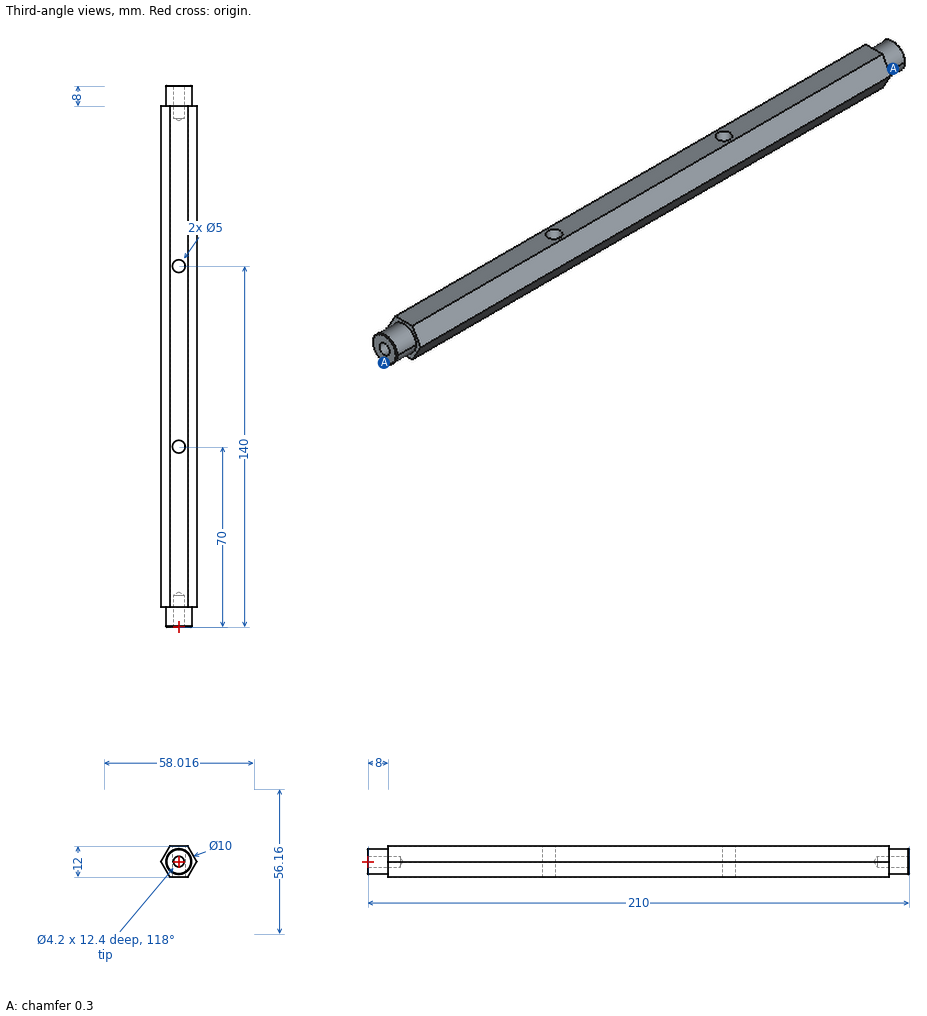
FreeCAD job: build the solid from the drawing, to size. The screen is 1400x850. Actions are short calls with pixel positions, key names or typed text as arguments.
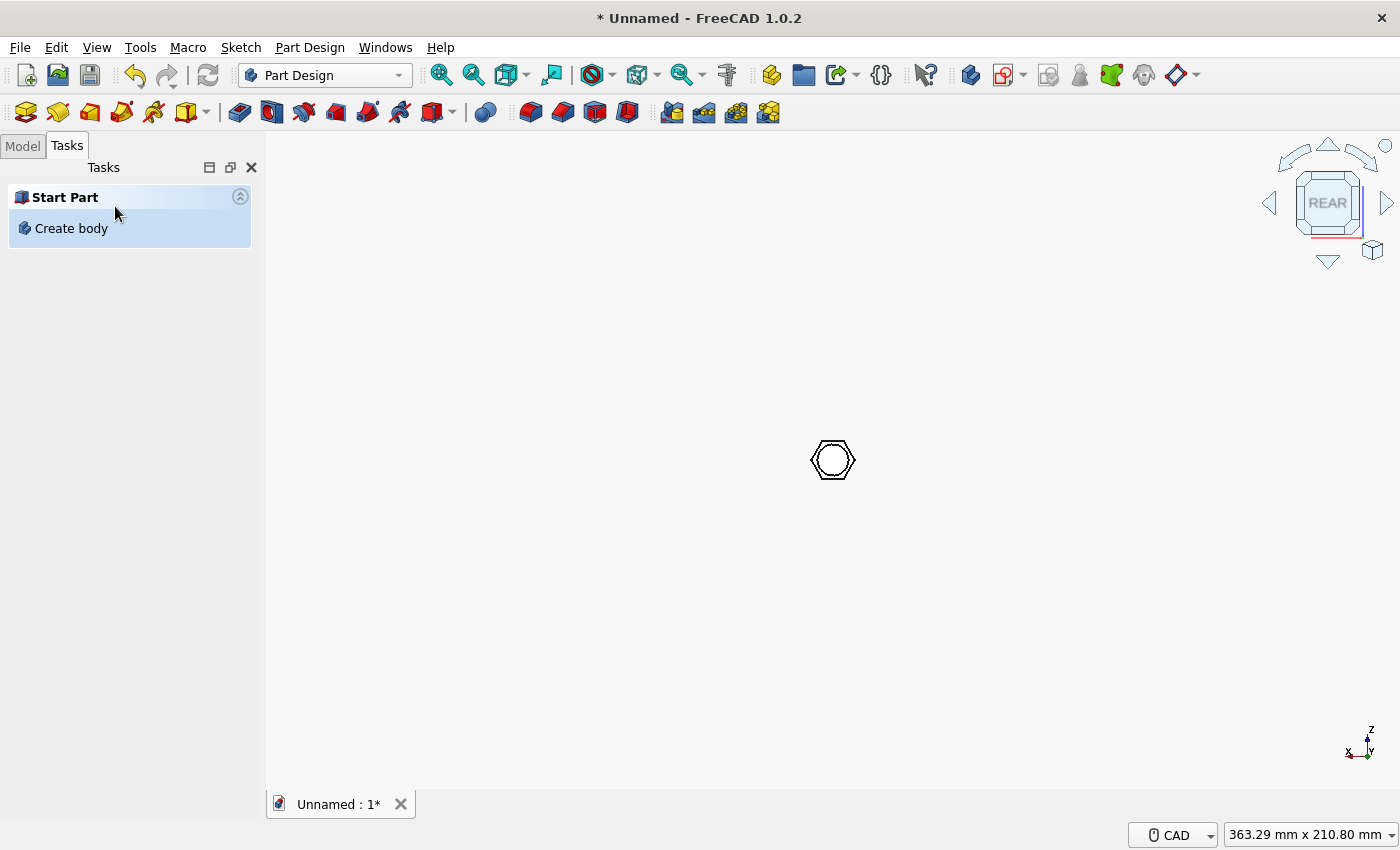
key(5)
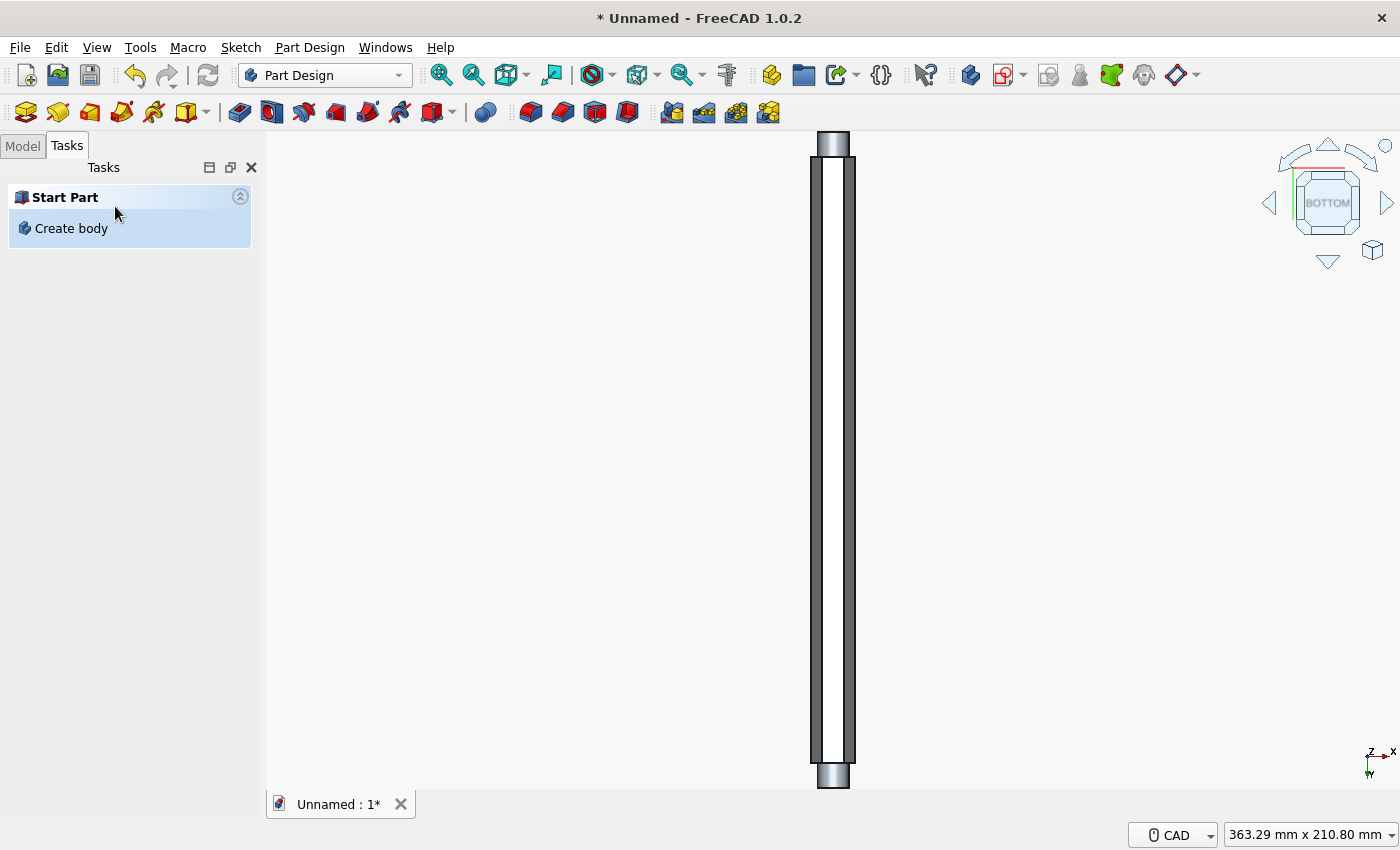
click(833, 719)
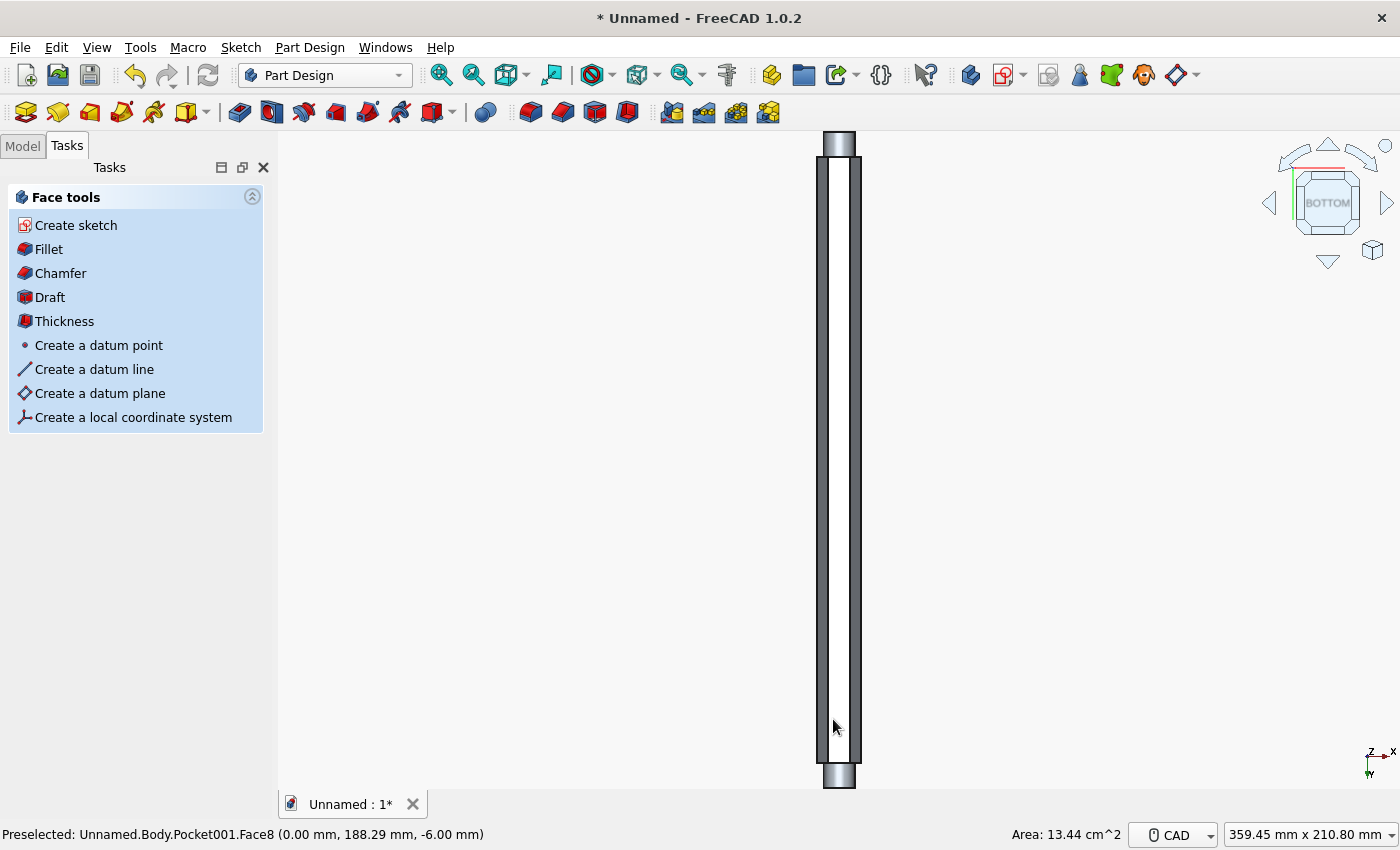
click(1004, 76)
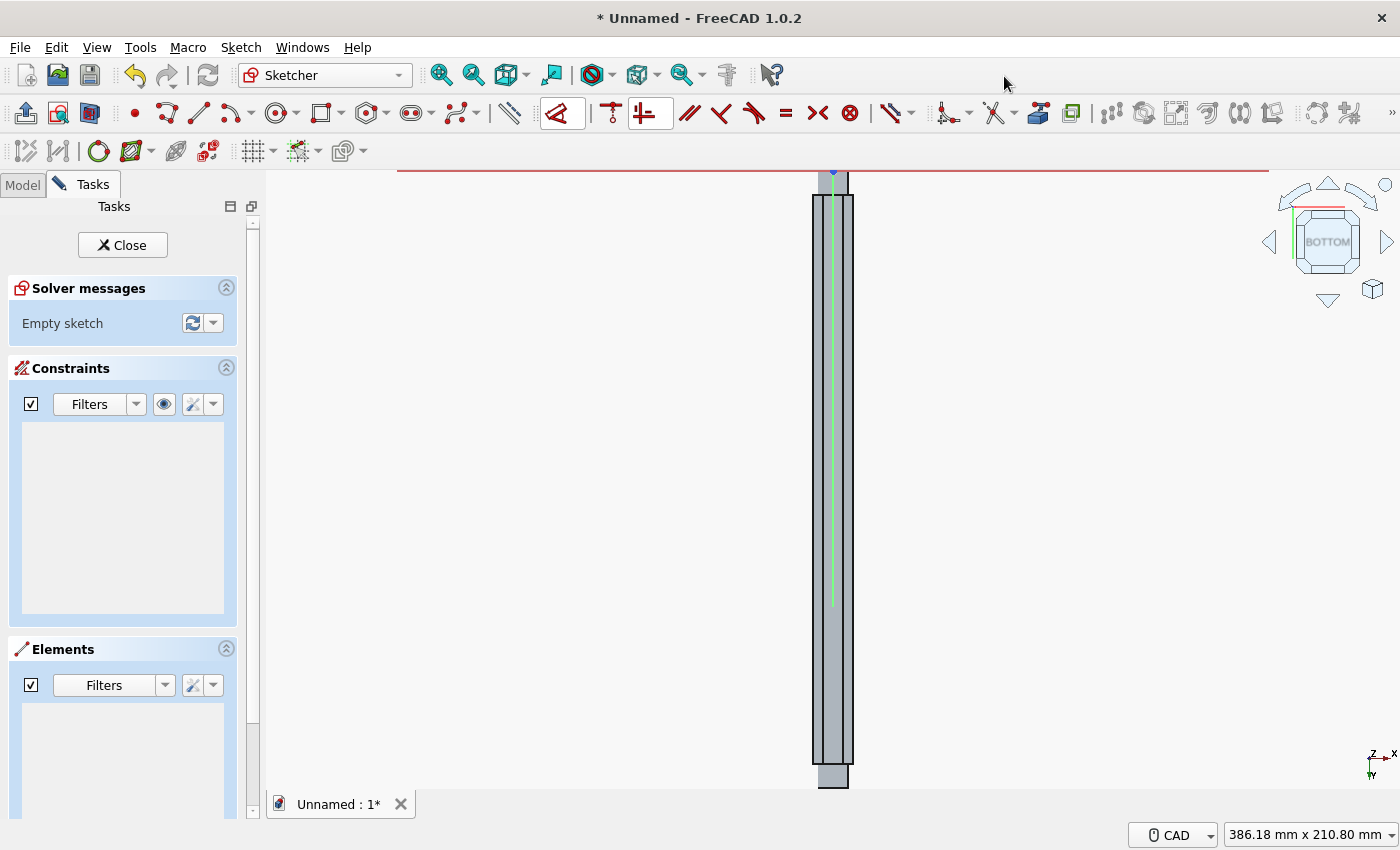
scroll(455, 761, down, 1)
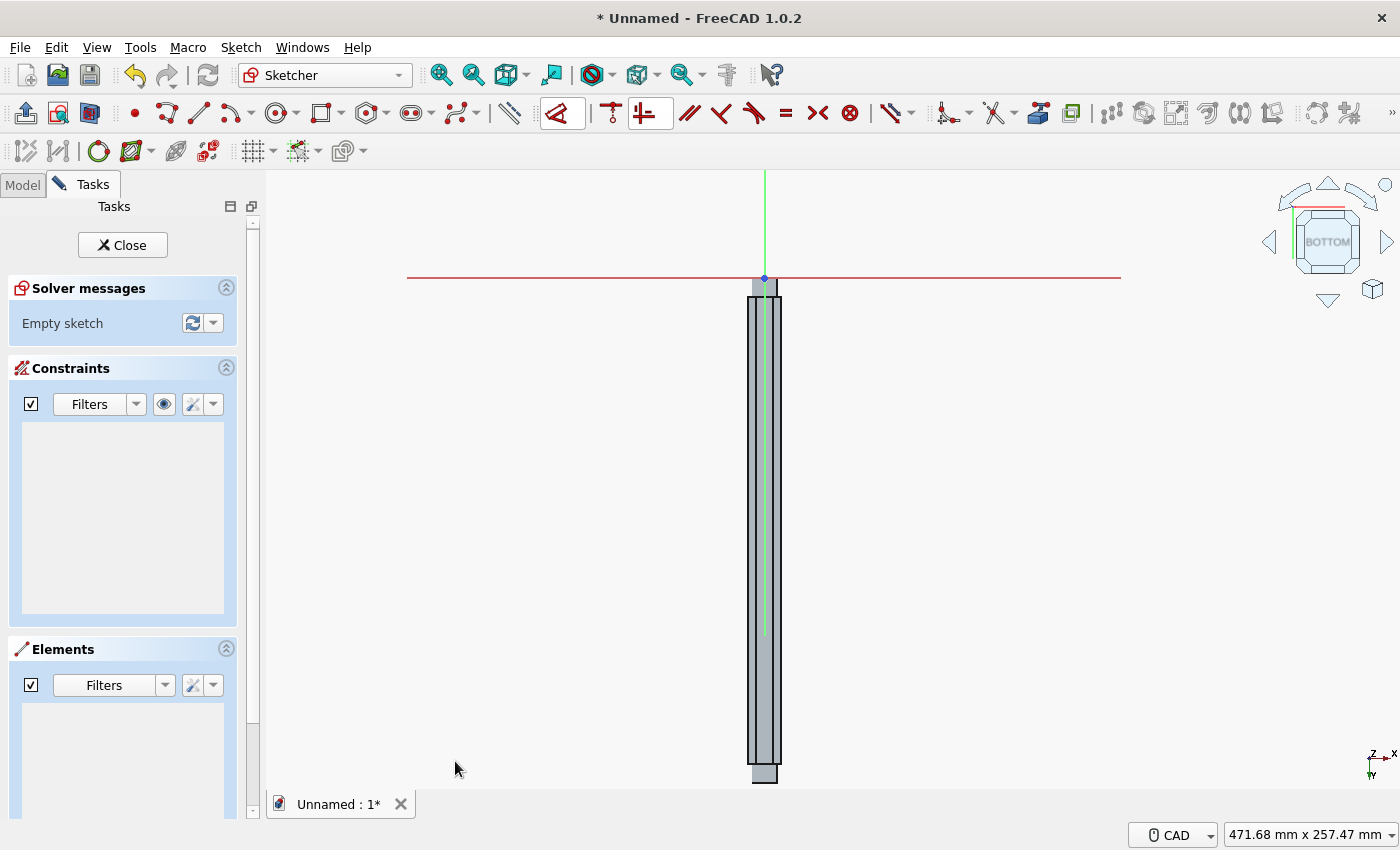
key(g)
key(c)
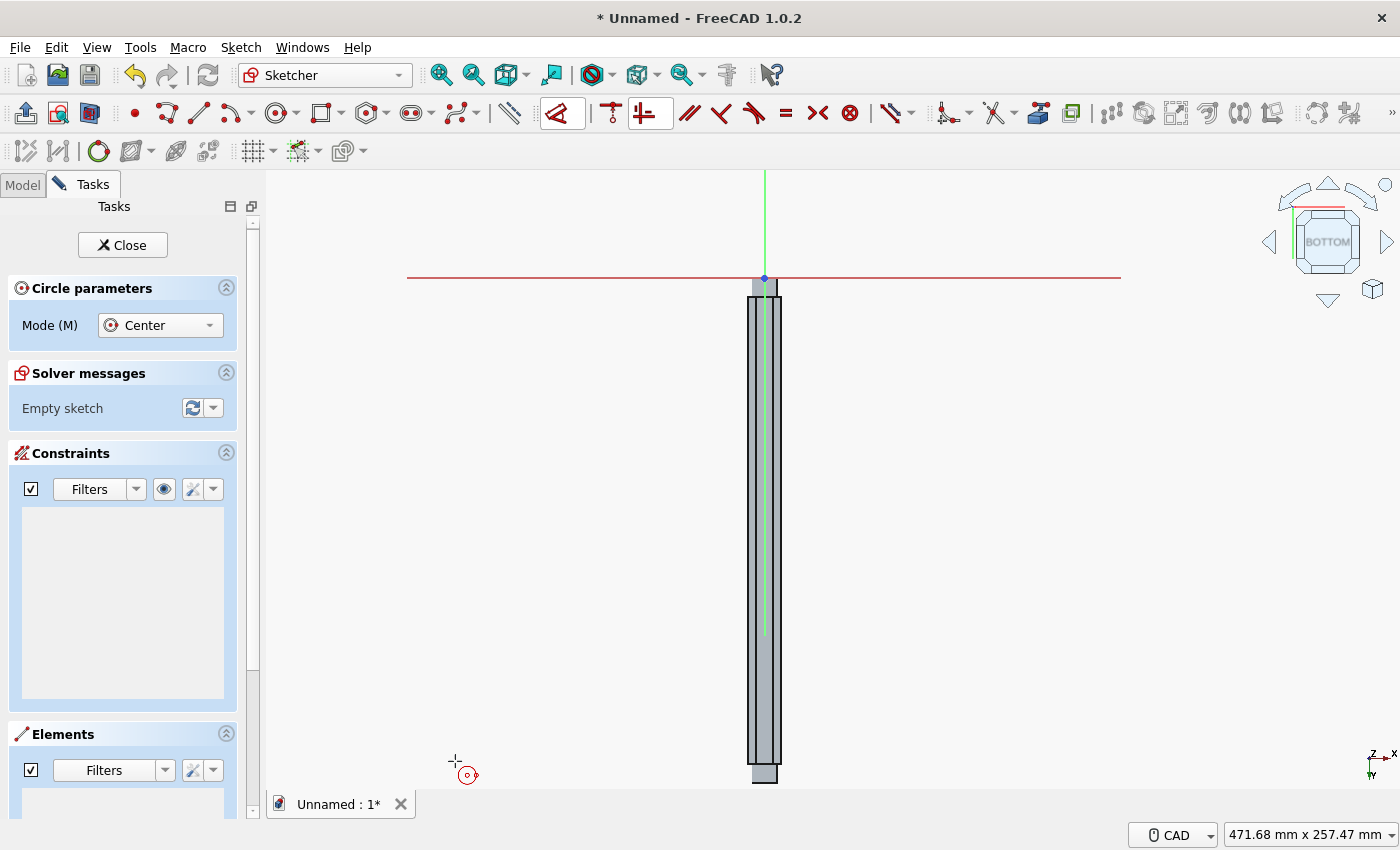
scroll(765, 615, up, 7)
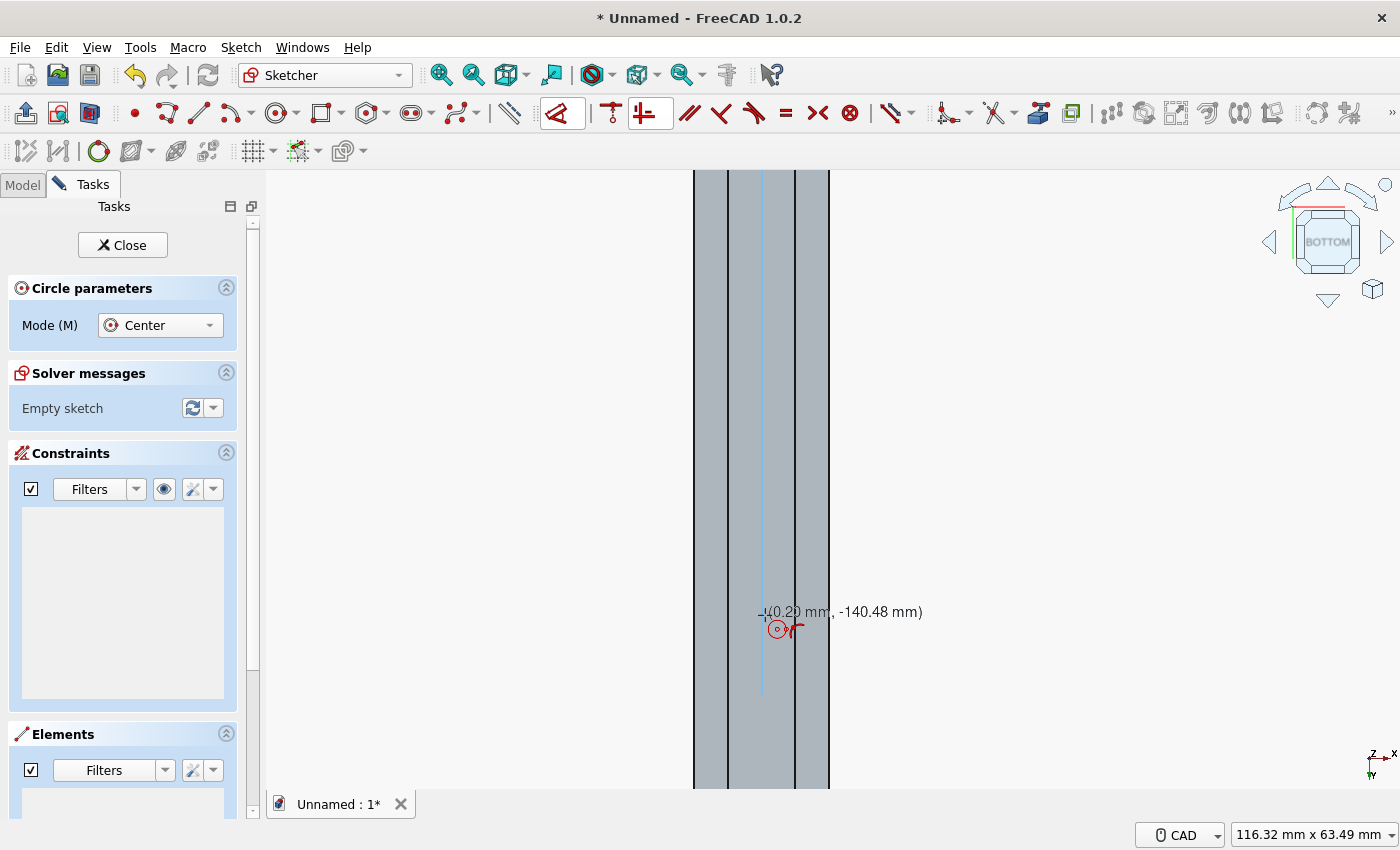
scroll(766, 711, down, 6)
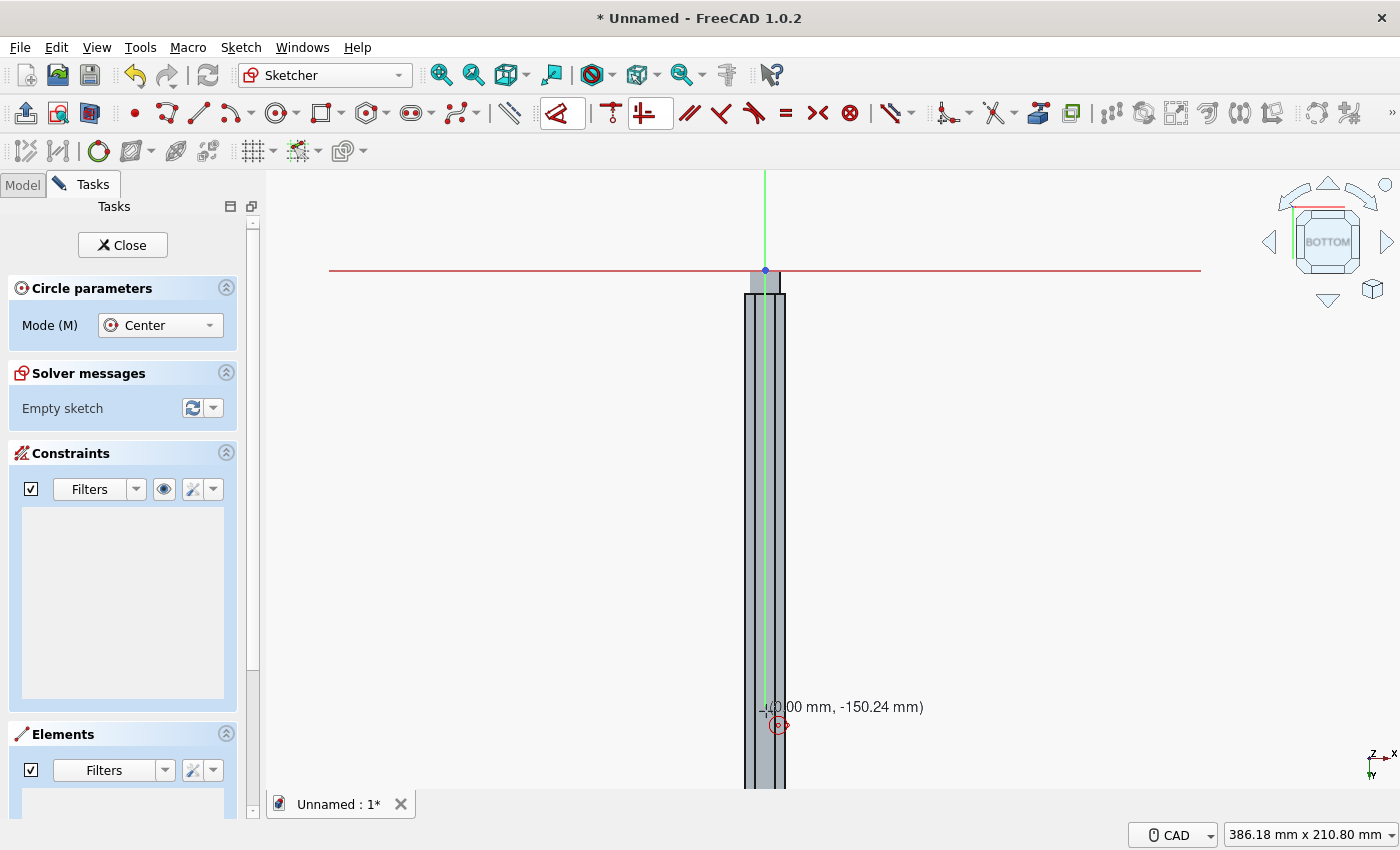
click(765, 682)